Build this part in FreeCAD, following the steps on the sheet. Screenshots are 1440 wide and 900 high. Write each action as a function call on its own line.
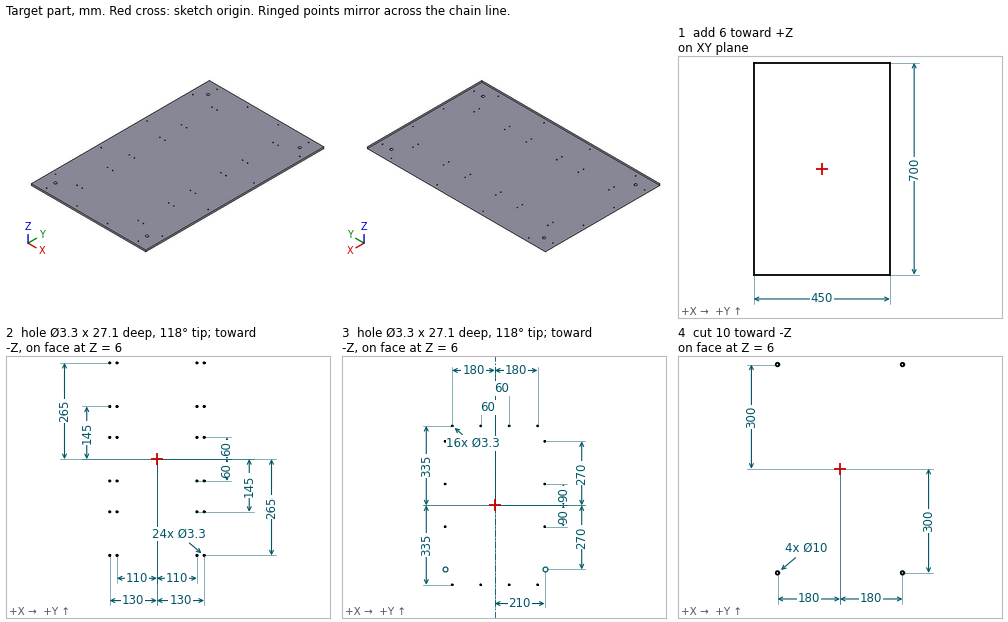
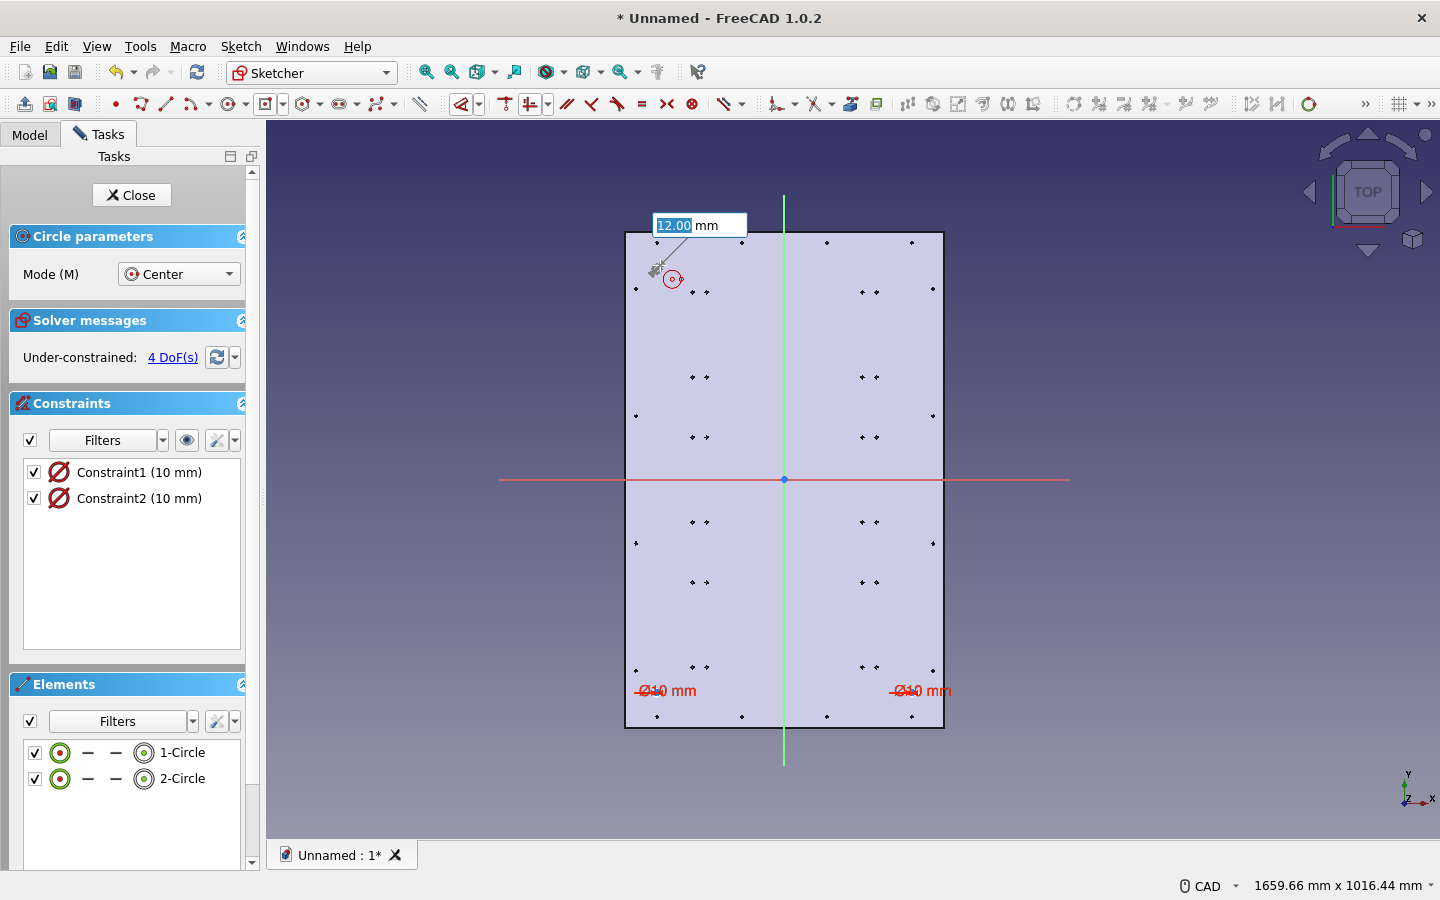
text(10)
key(Return)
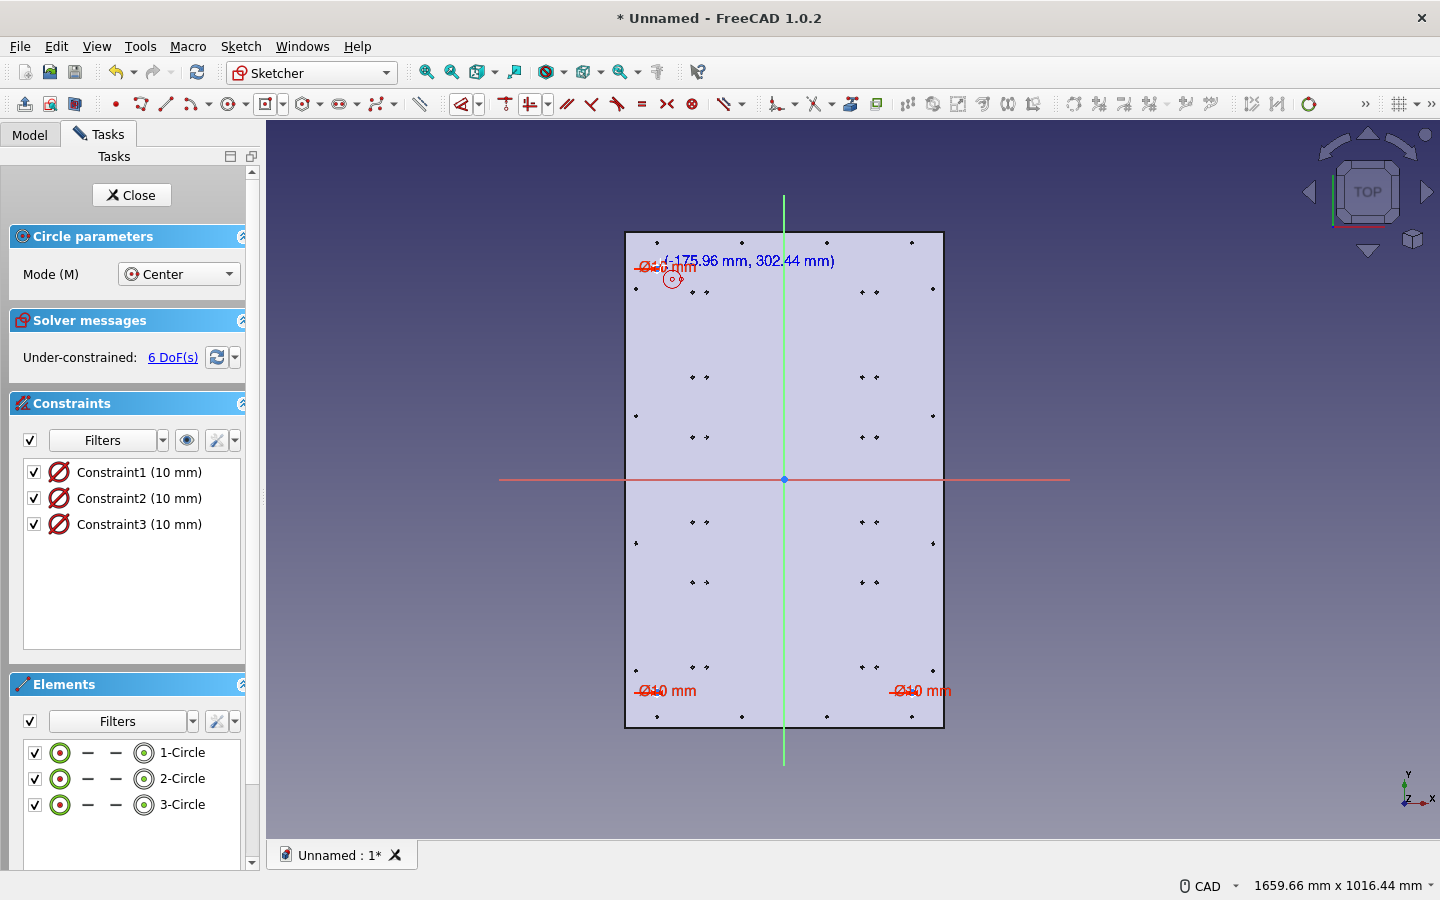
scroll(912, 268, up, 10)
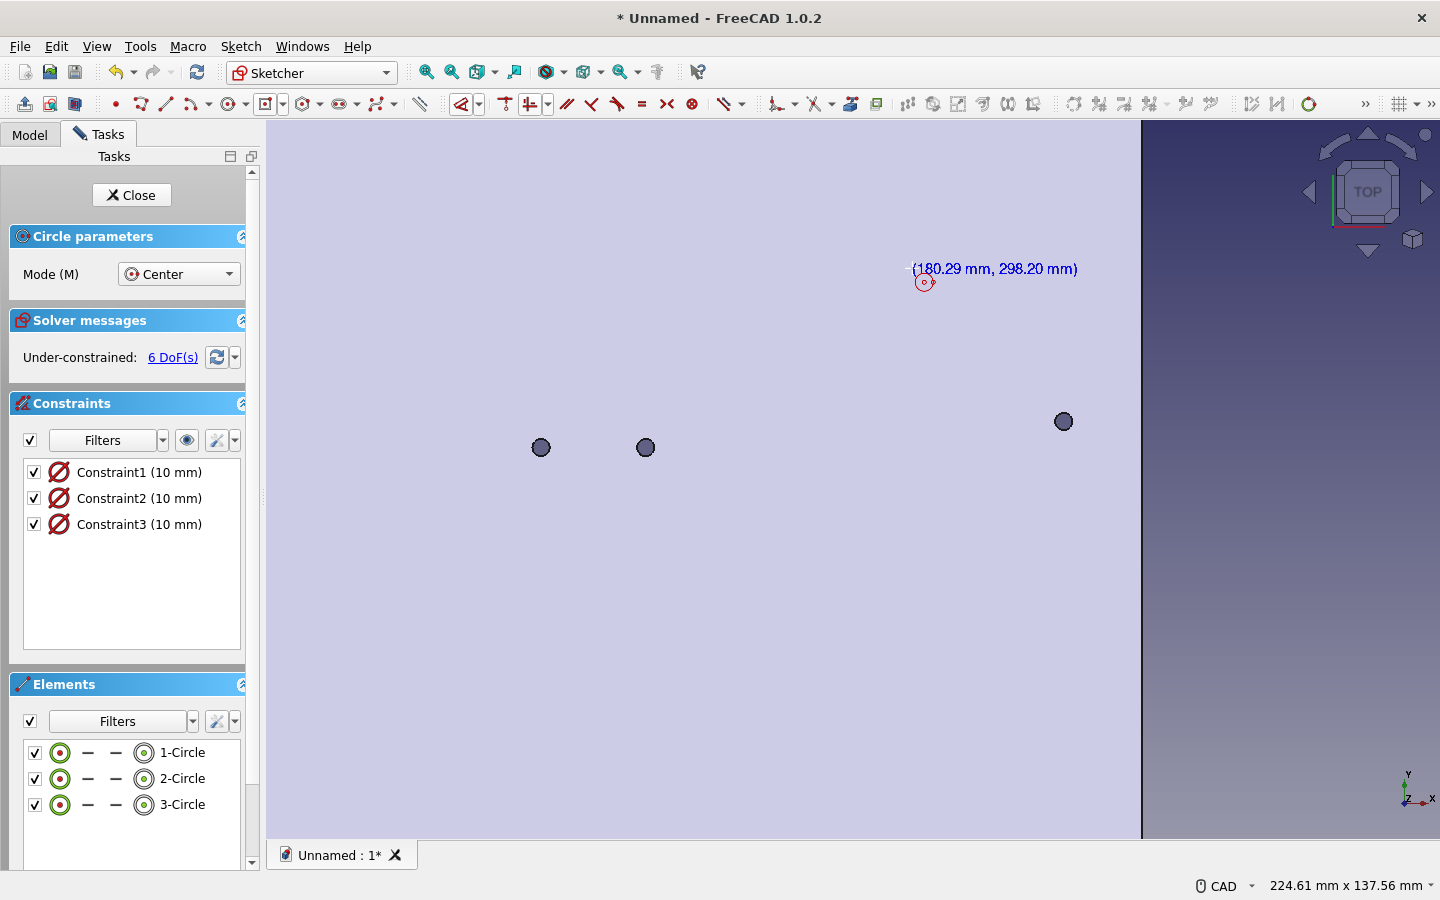
scroll(913, 268, down, 10)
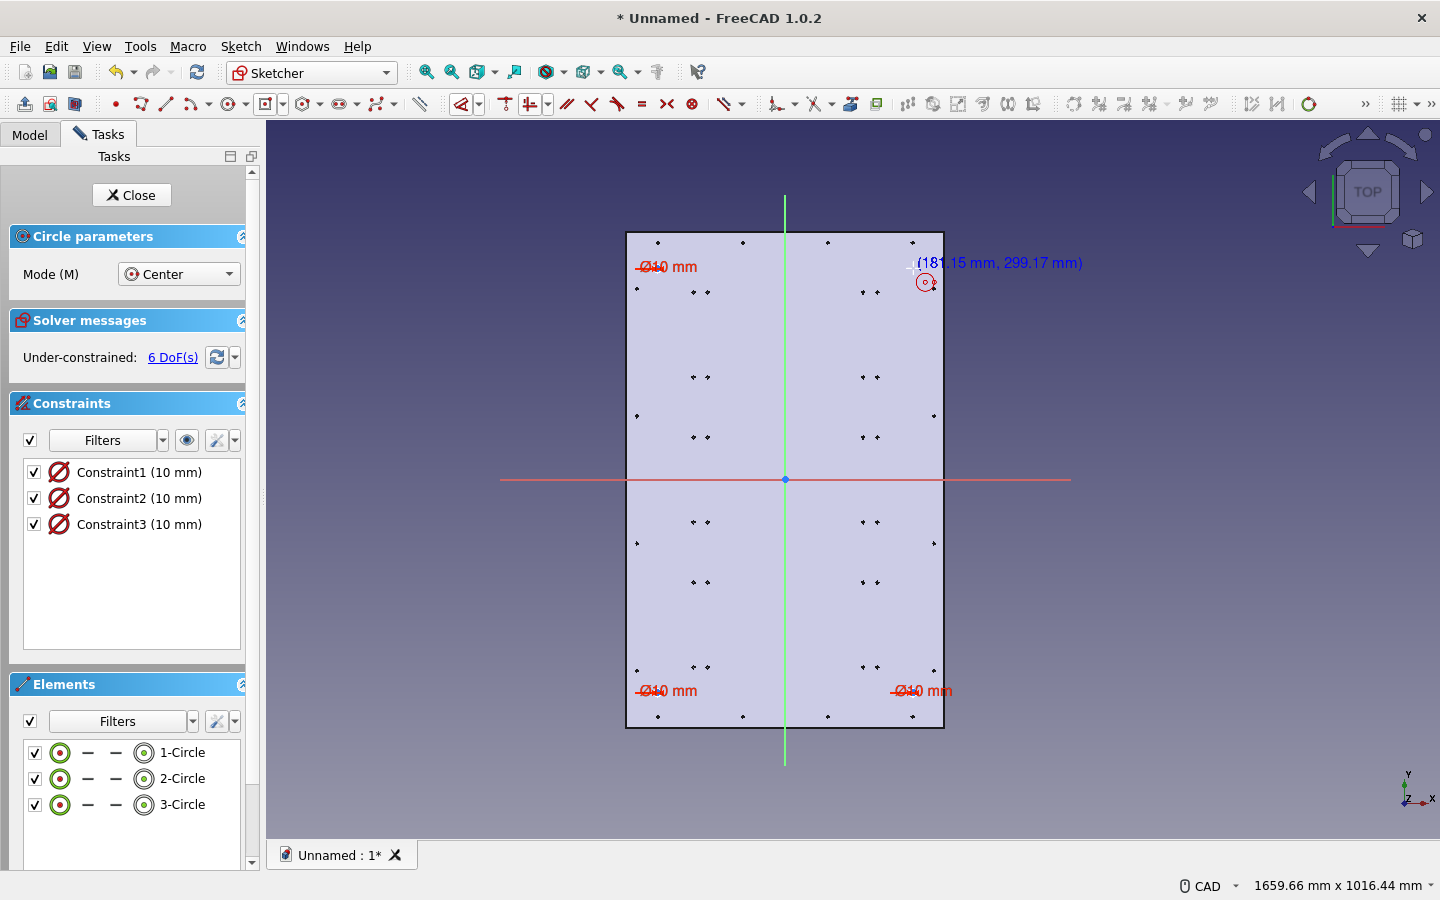
click(913, 268)
move(915, 265)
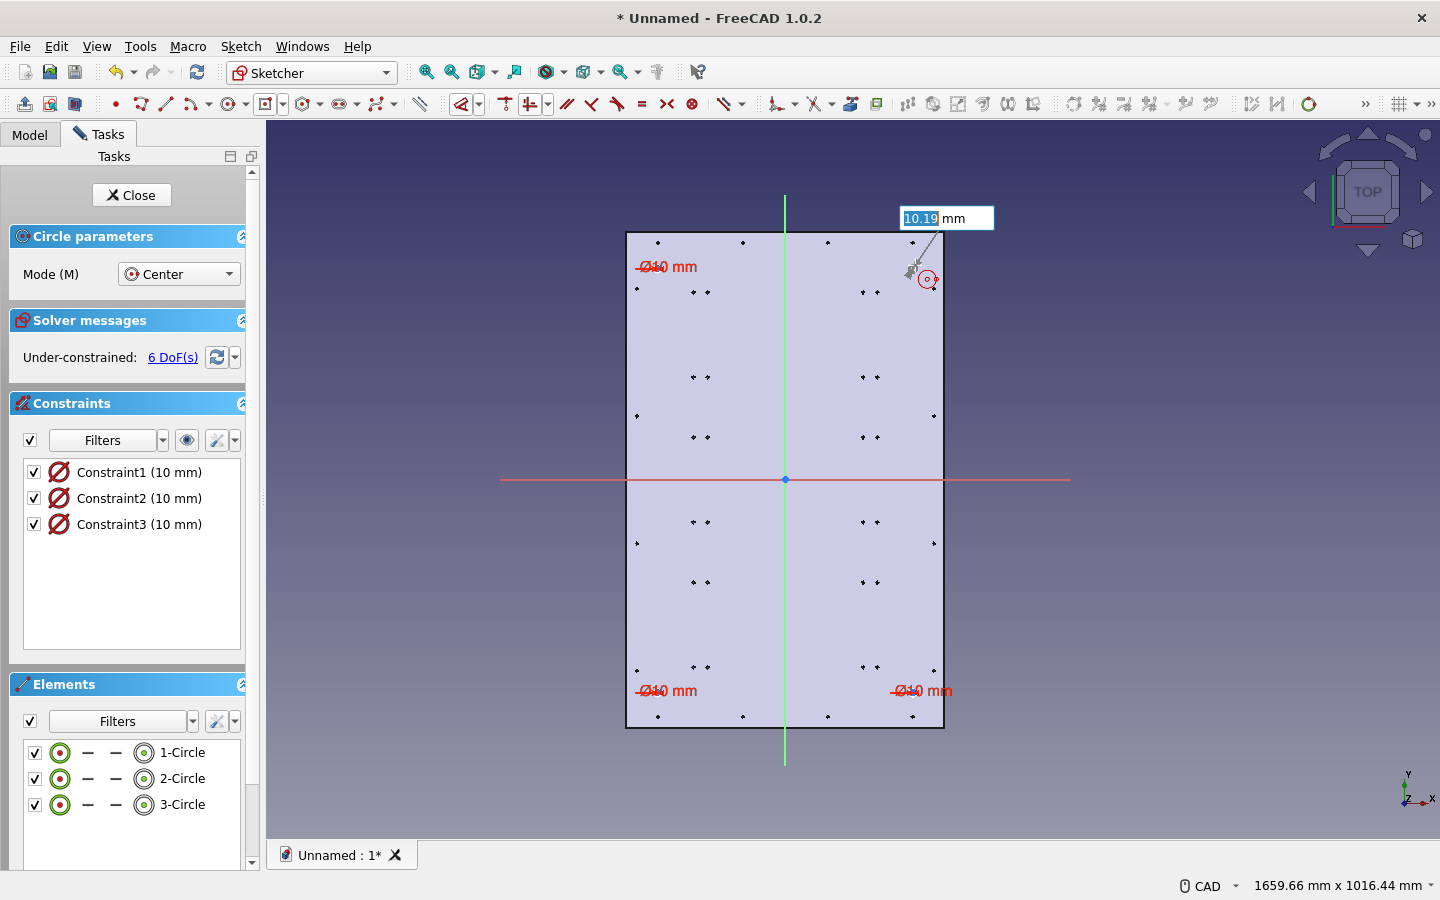
text(10)
key(Return)
key(Escape)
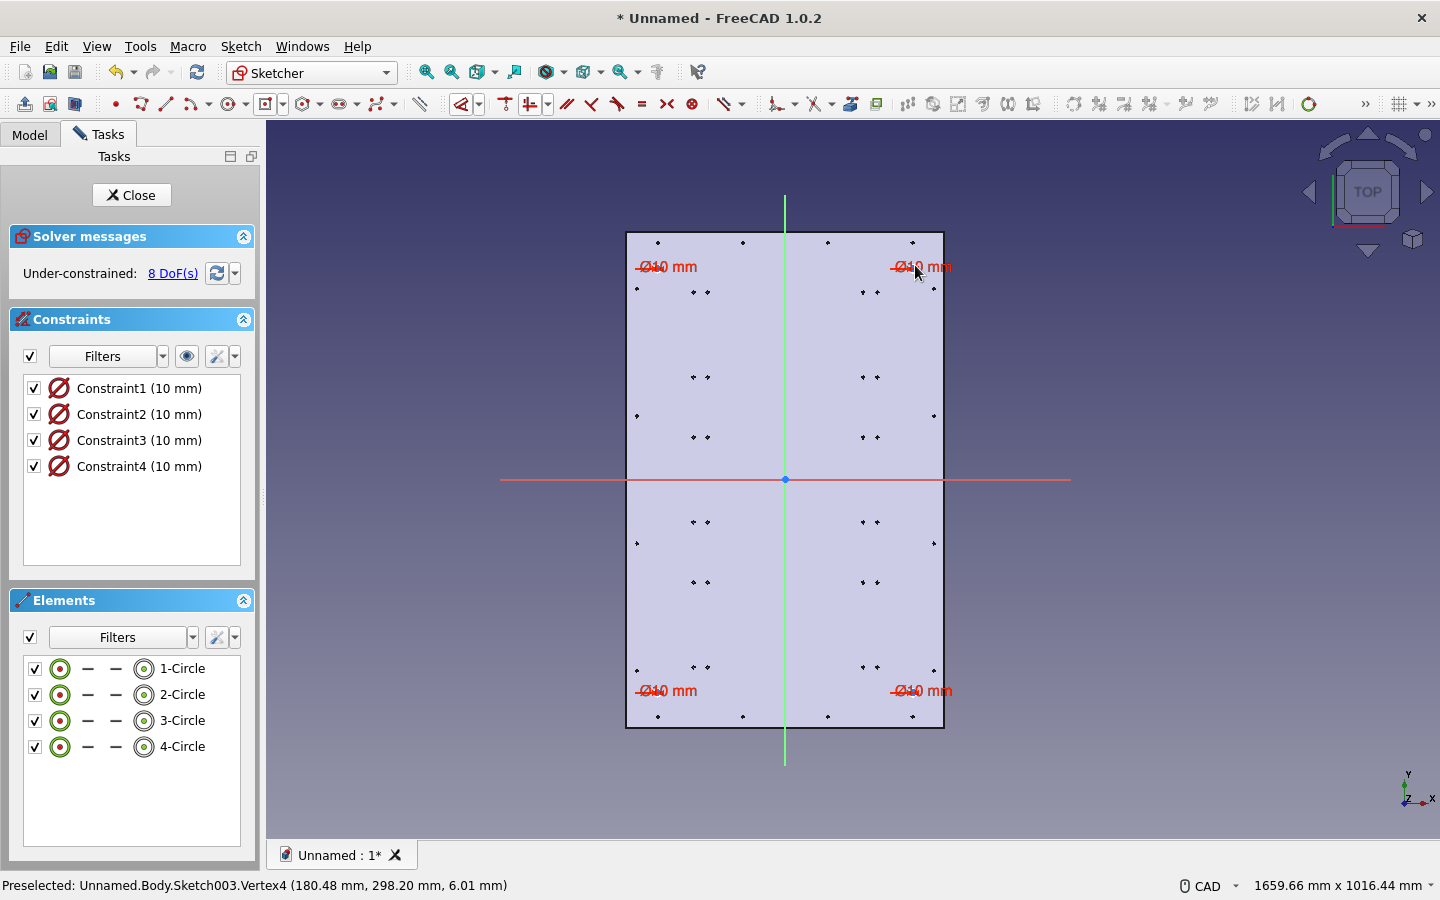
click(913, 693)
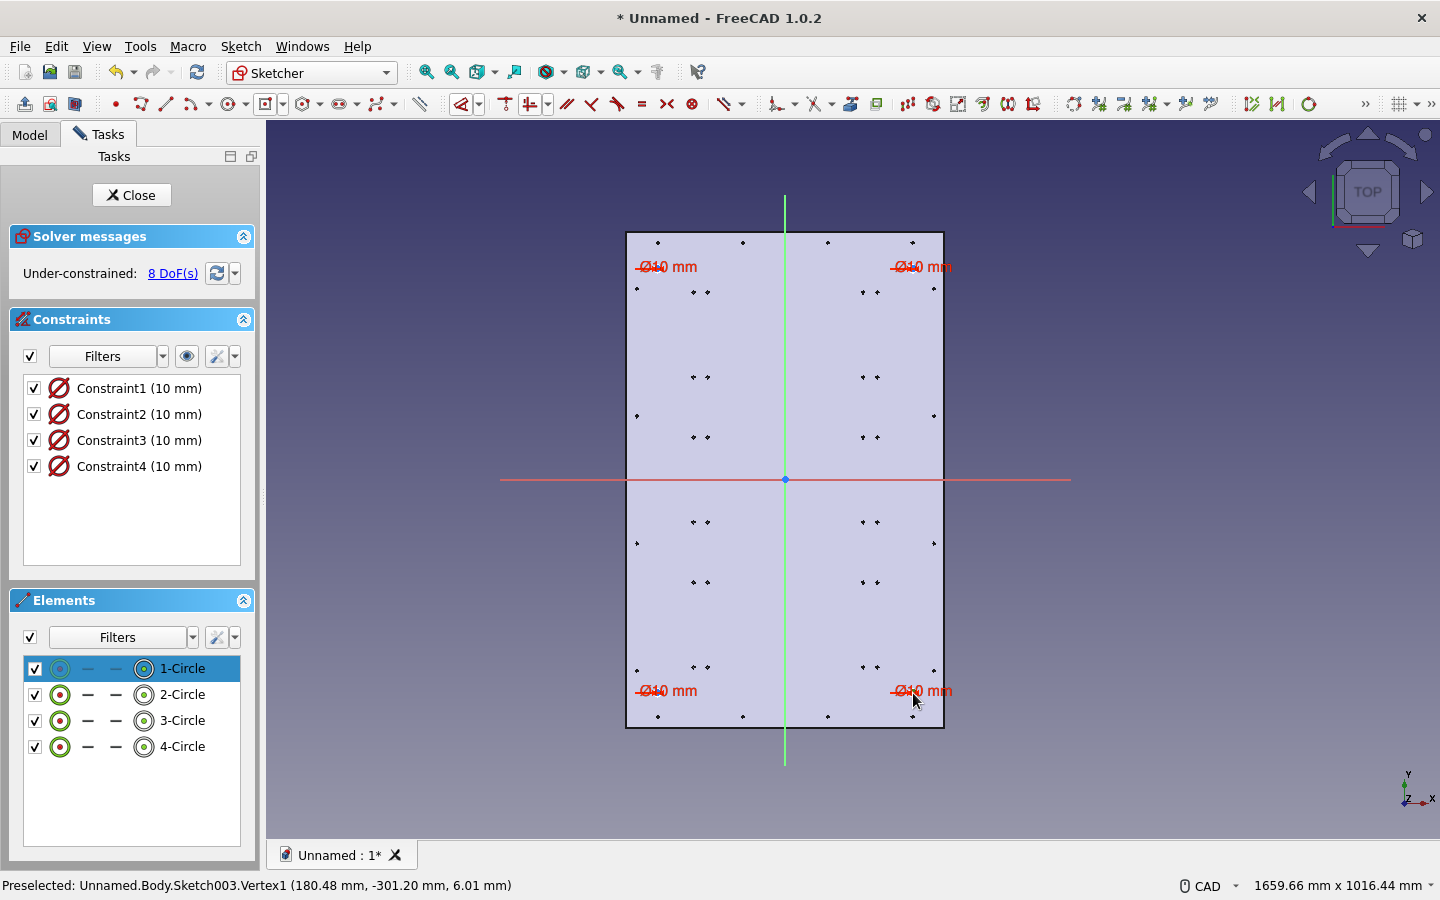
click(658, 693)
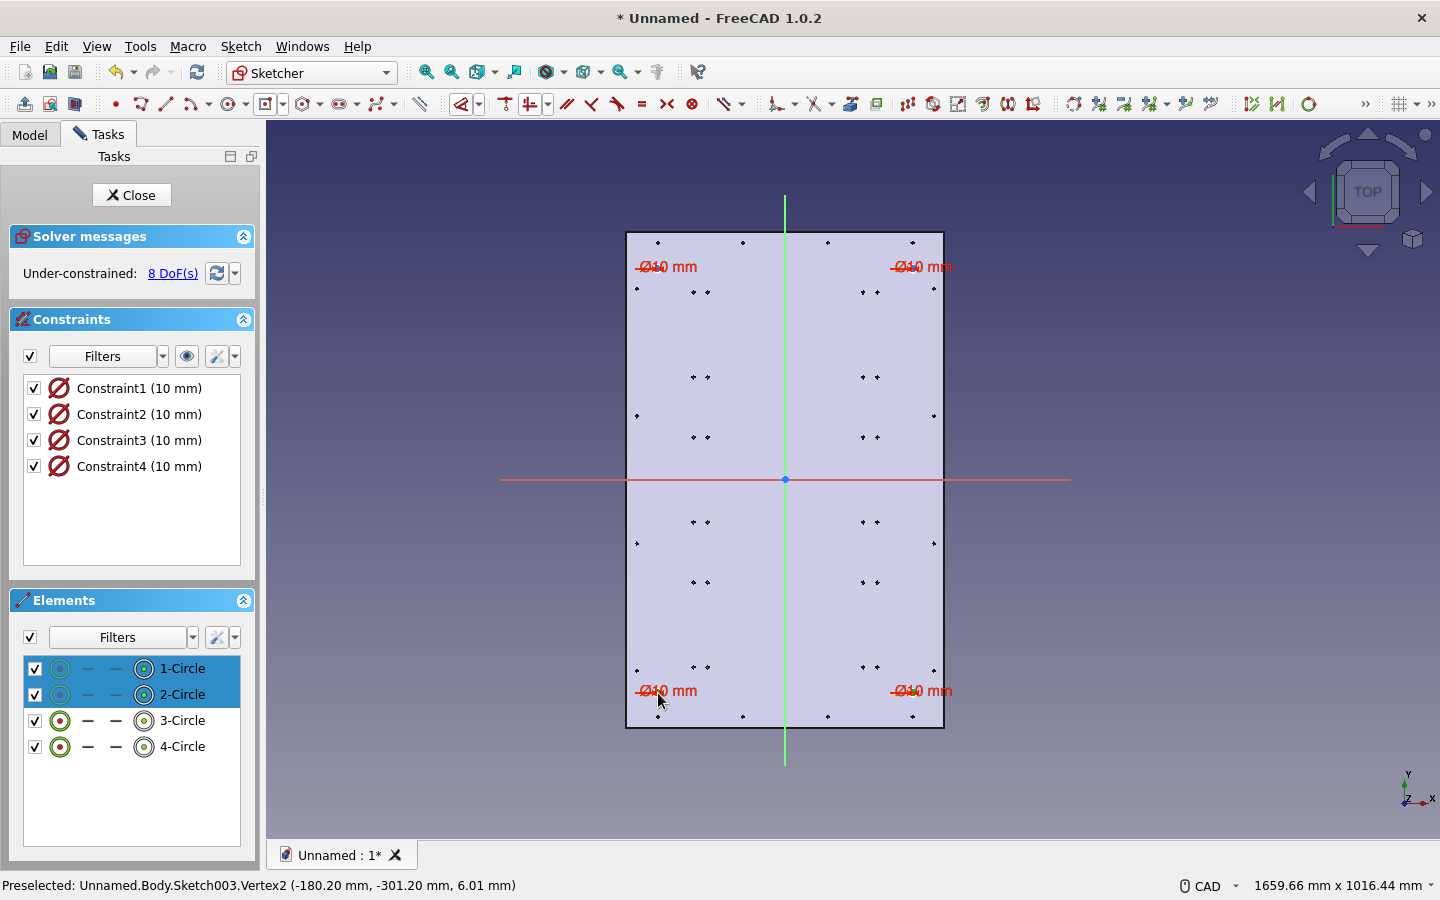
click(548, 104)